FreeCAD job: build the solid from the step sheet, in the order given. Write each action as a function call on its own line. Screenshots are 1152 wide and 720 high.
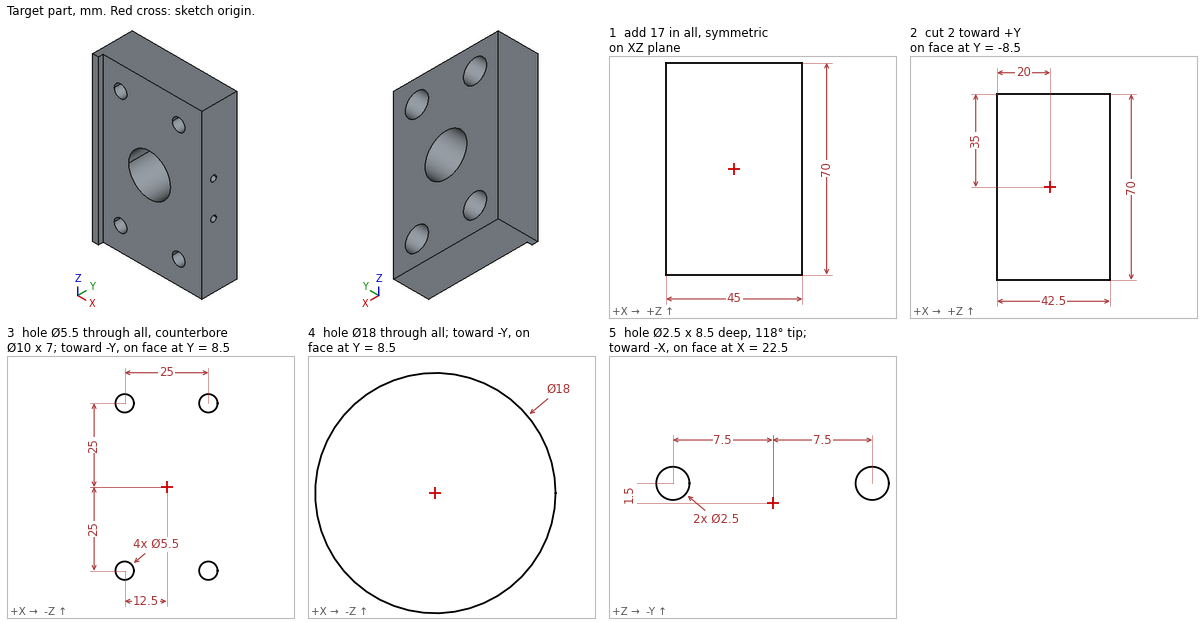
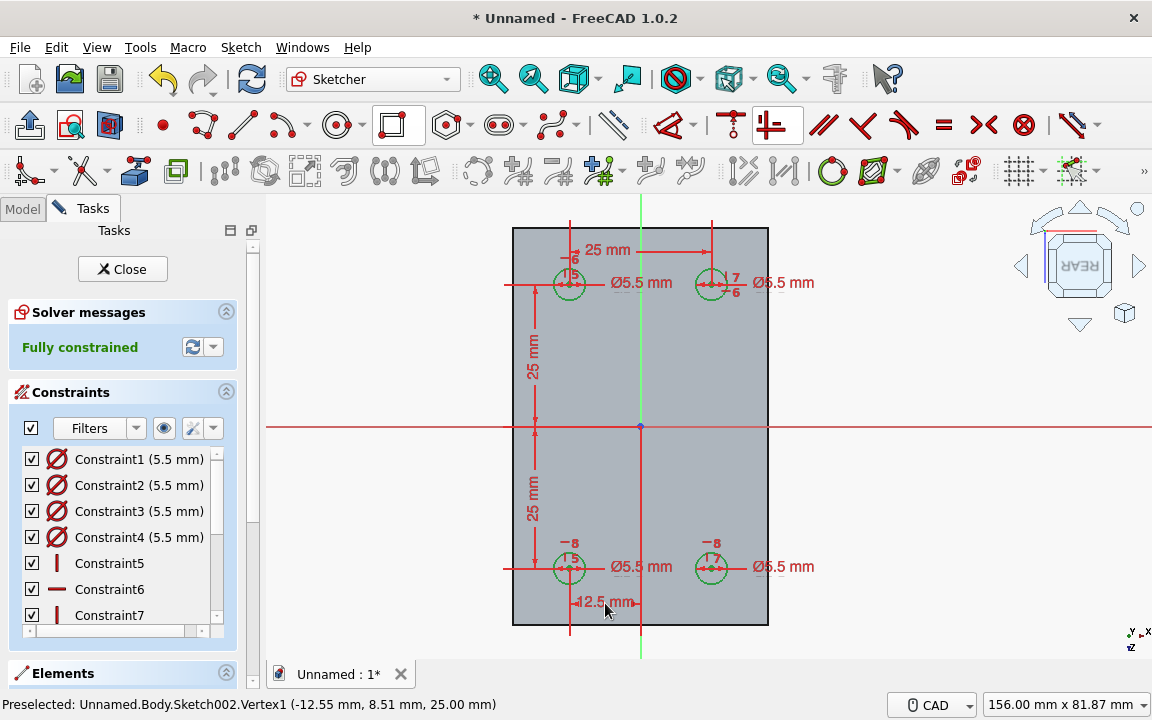
click(123, 269)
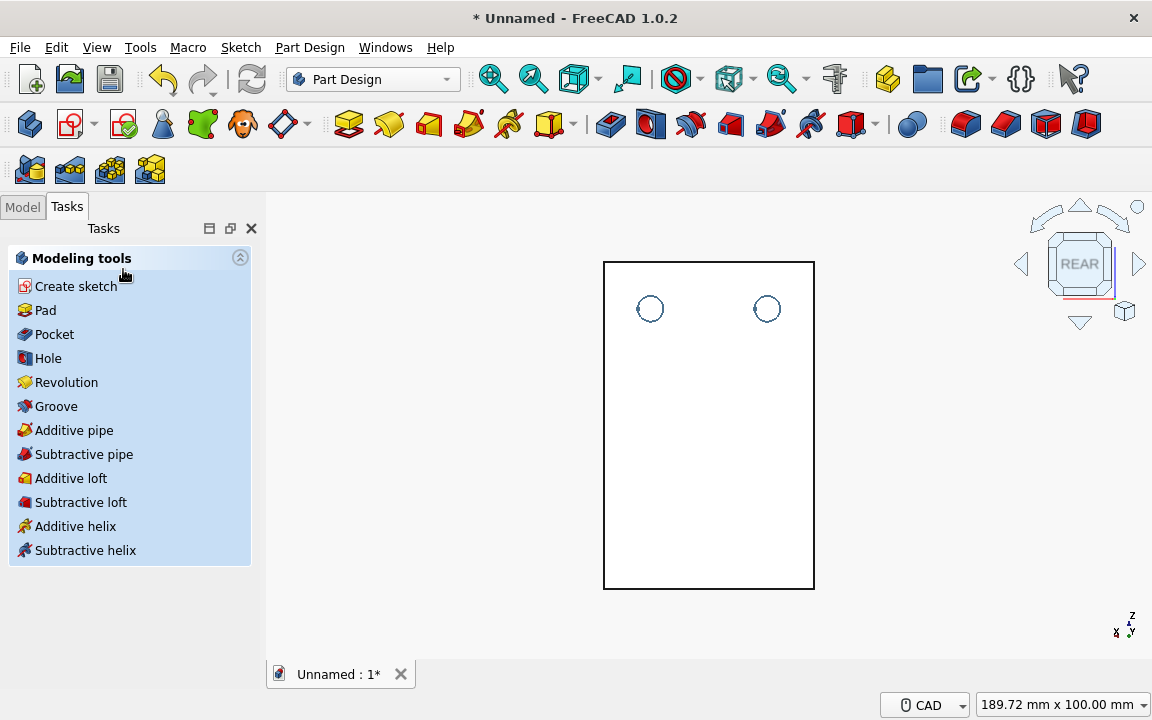
click(652, 124)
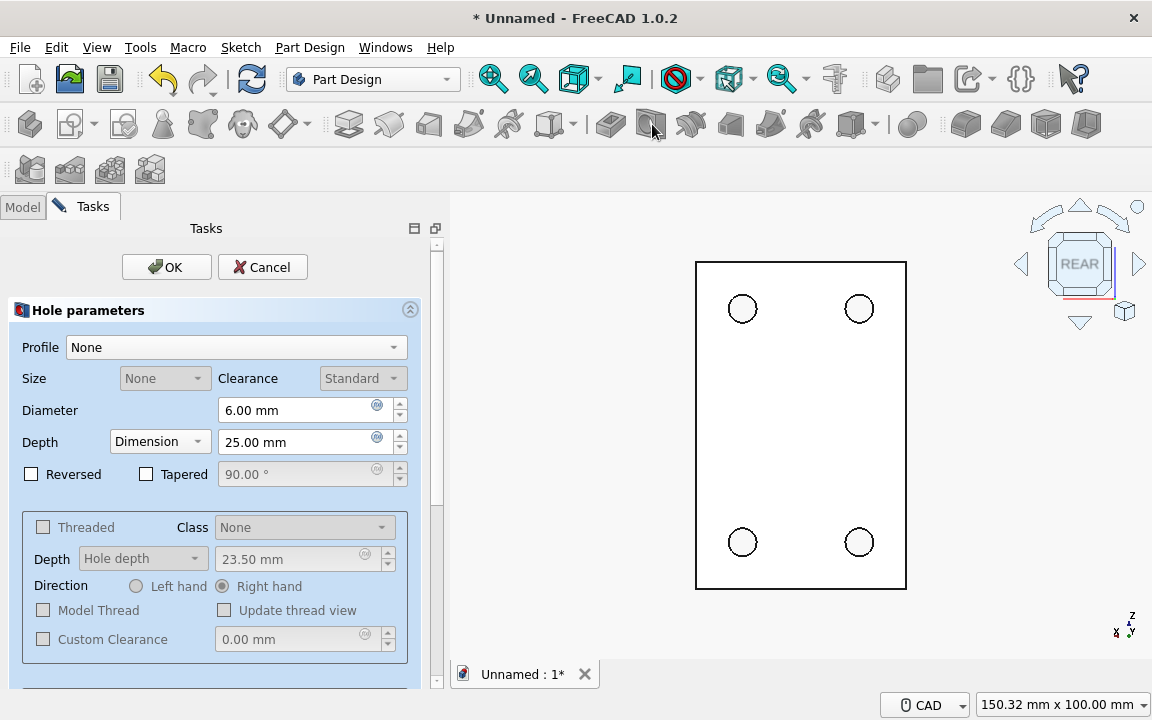
triple_click(305, 410)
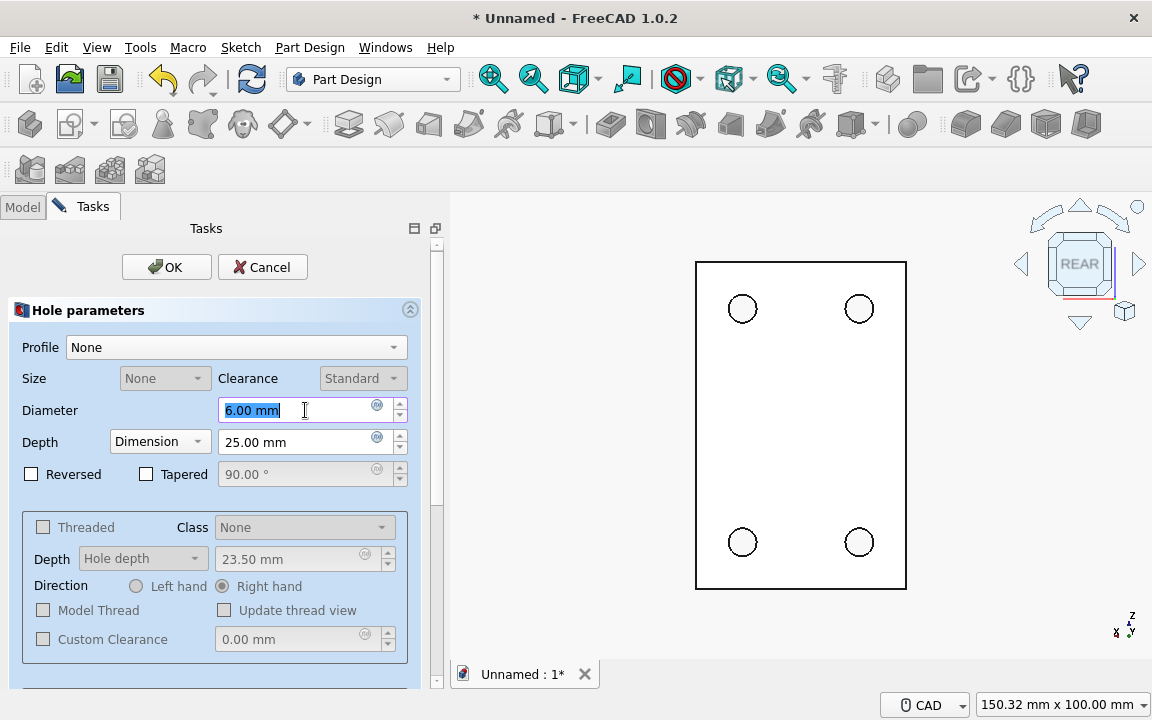
text(5.5)
key(Tab)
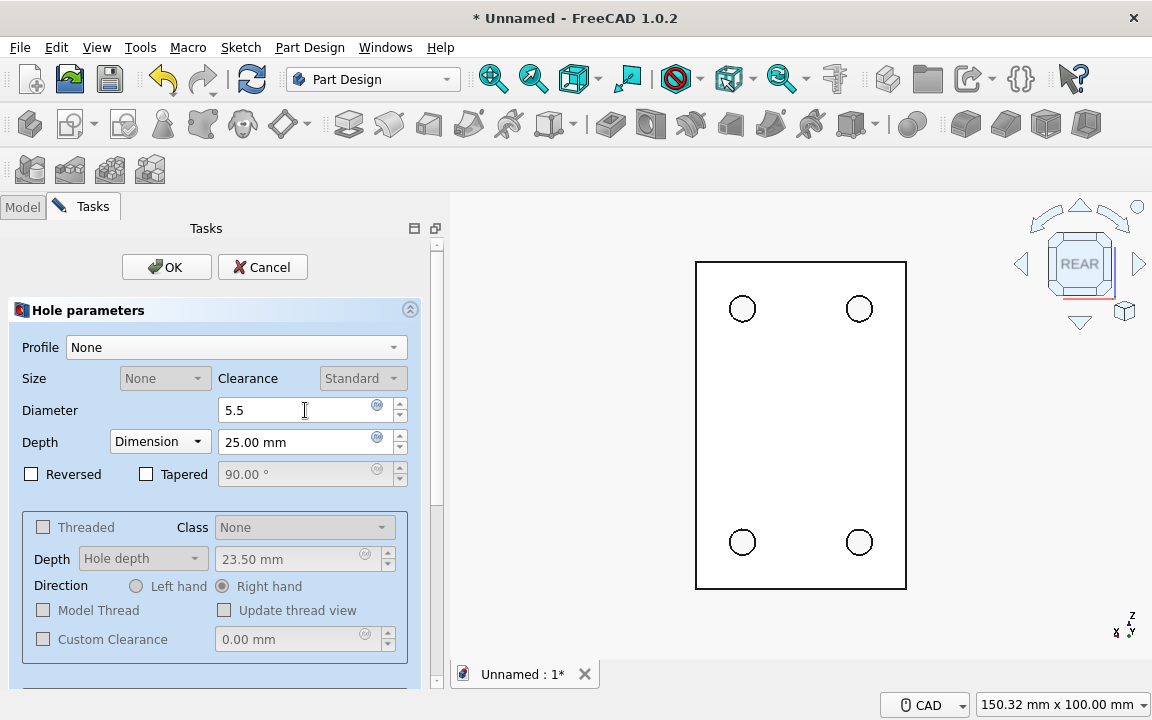
click(161, 442)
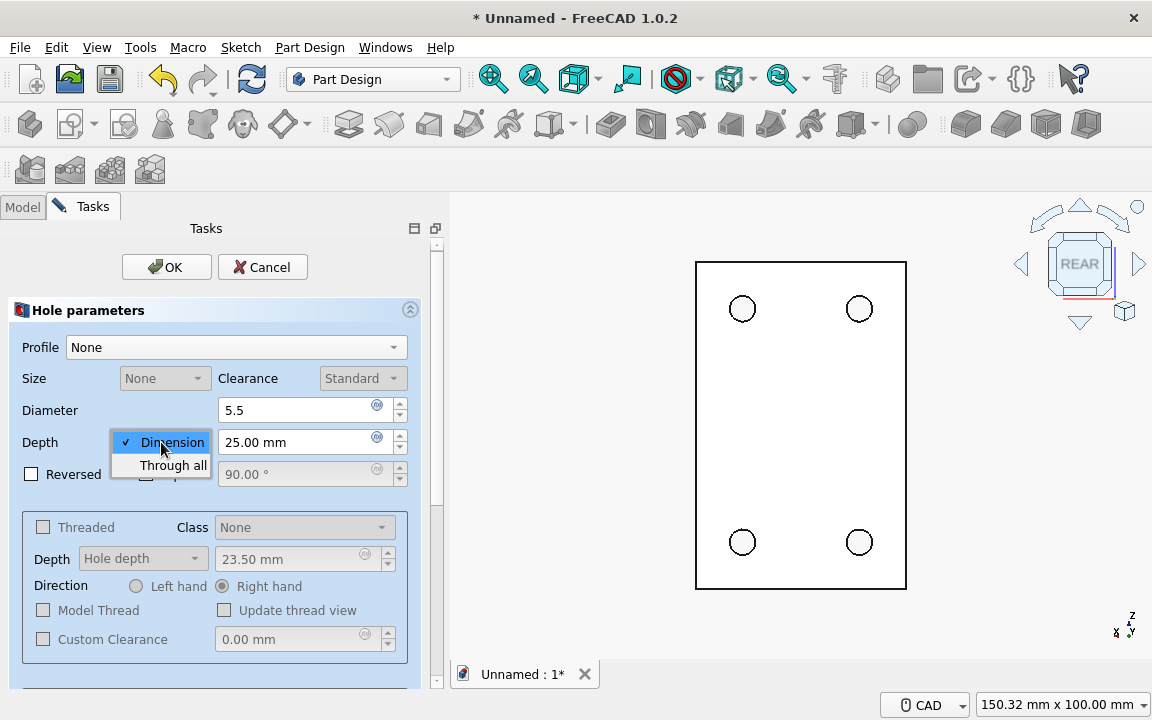
click(160, 466)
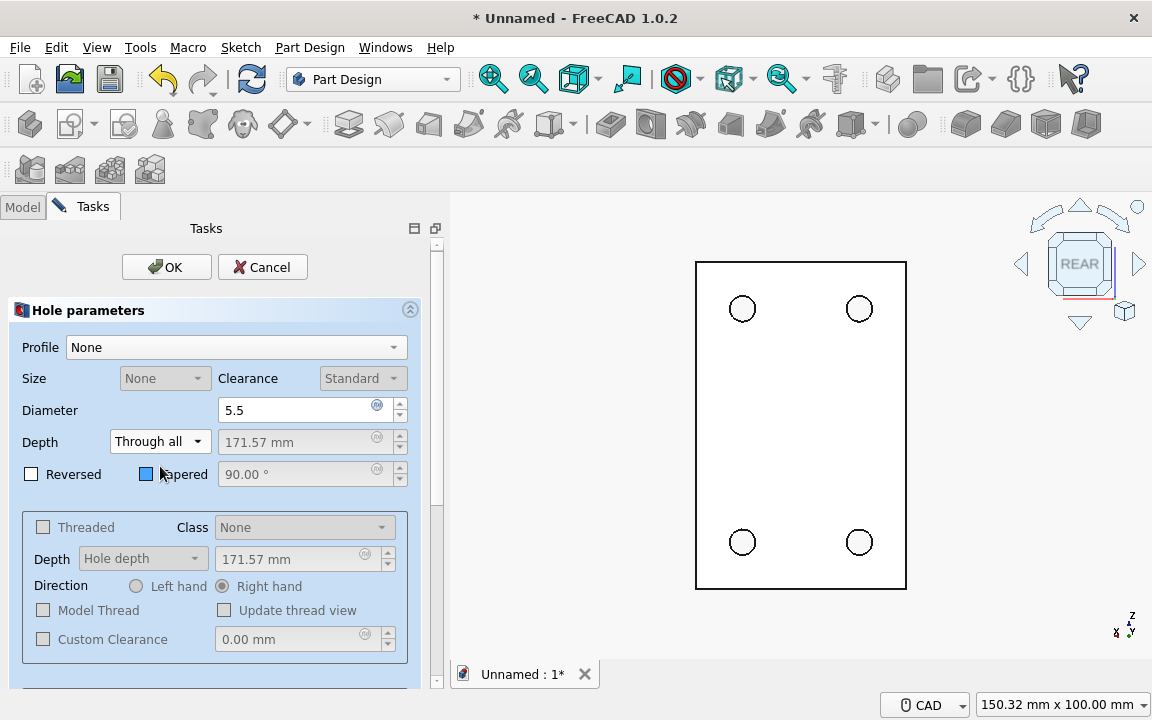
scroll(437, 463, down, 2)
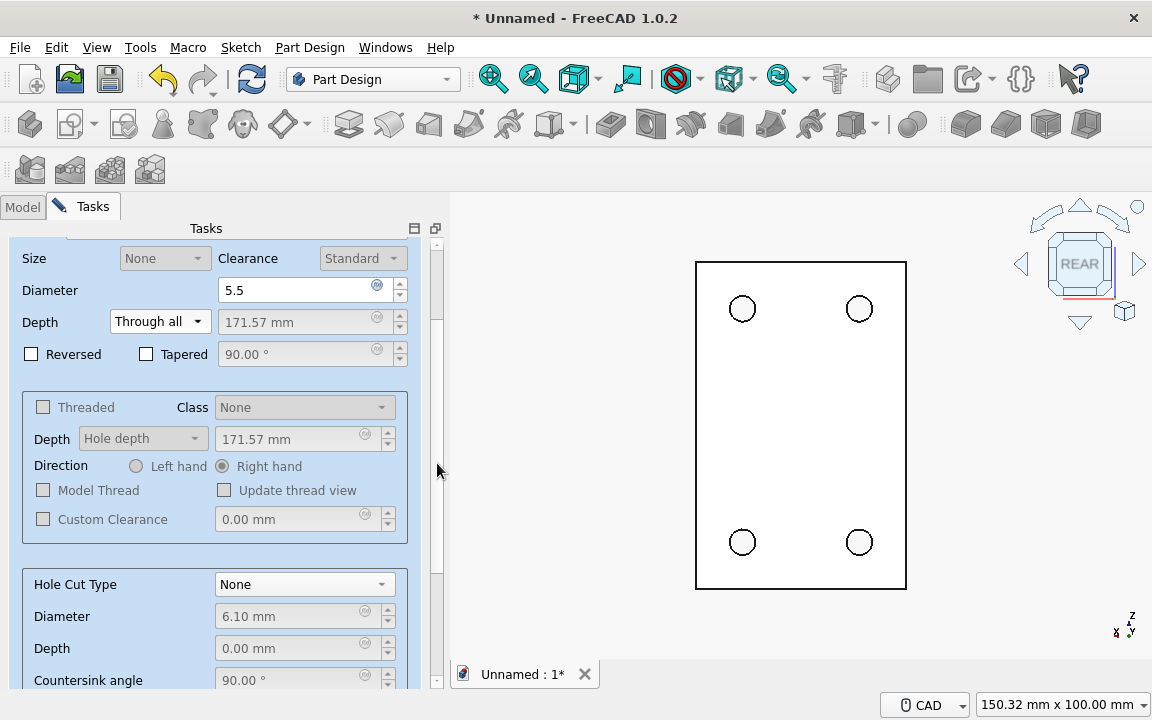
click(306, 584)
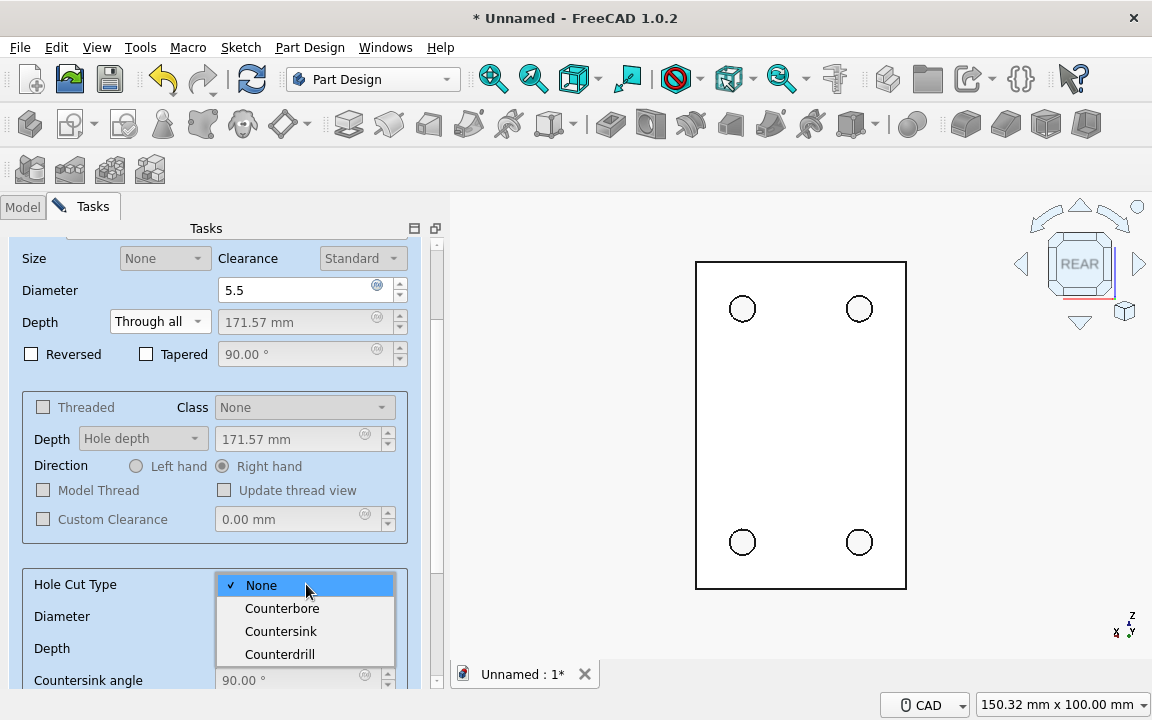
click(304, 608)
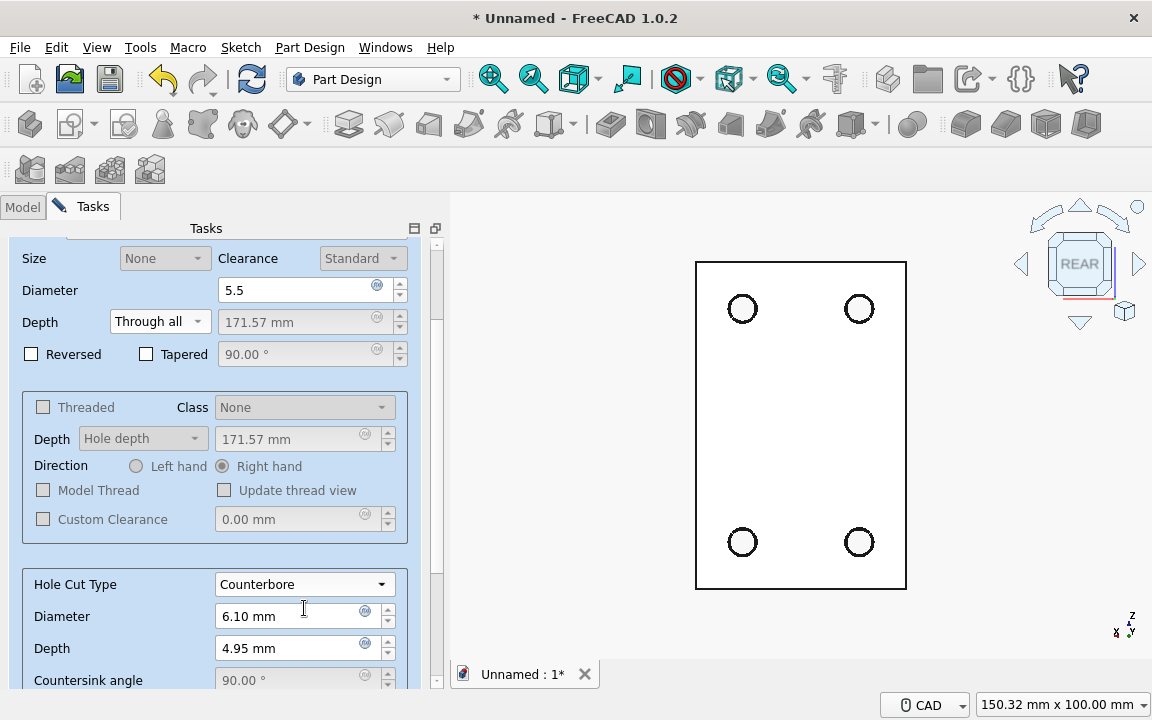
triple_click(298, 616)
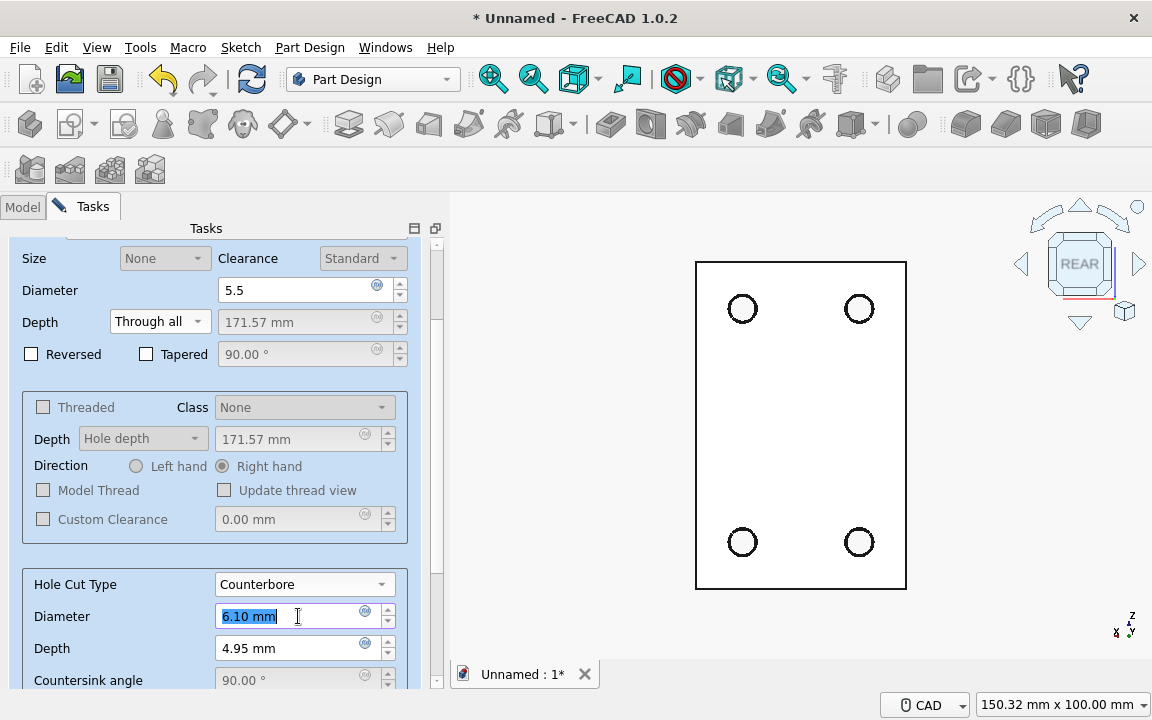
text(10)
key(Tab)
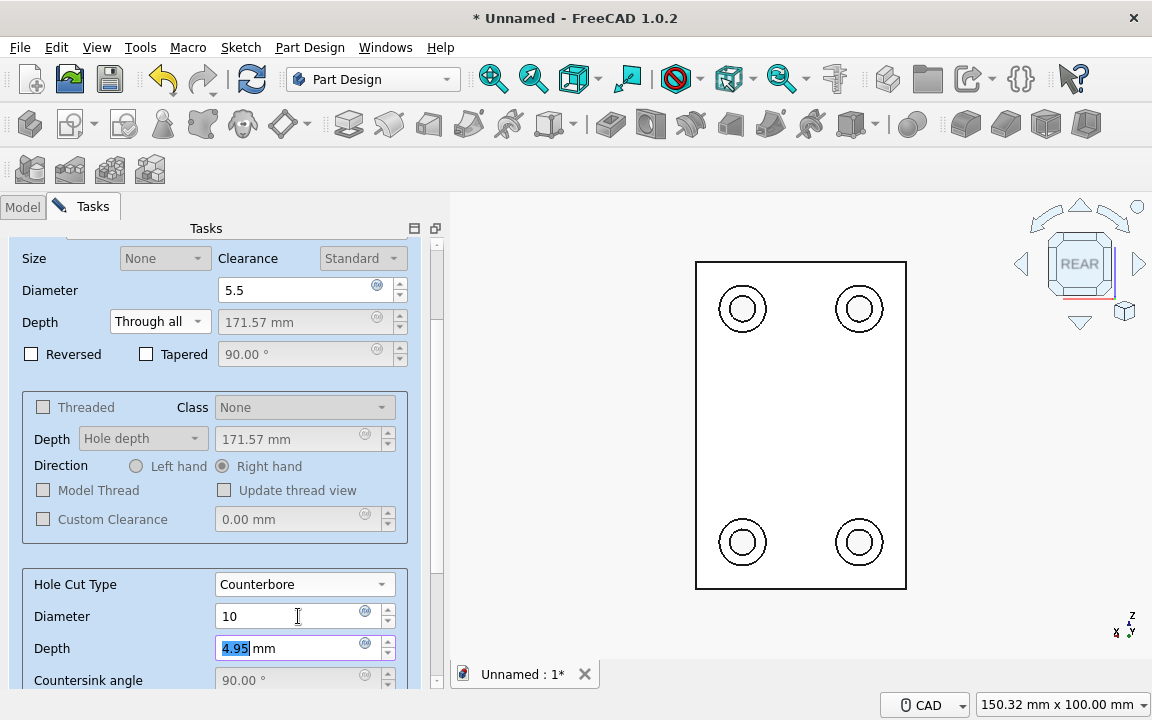
text(7)
key(Tab)